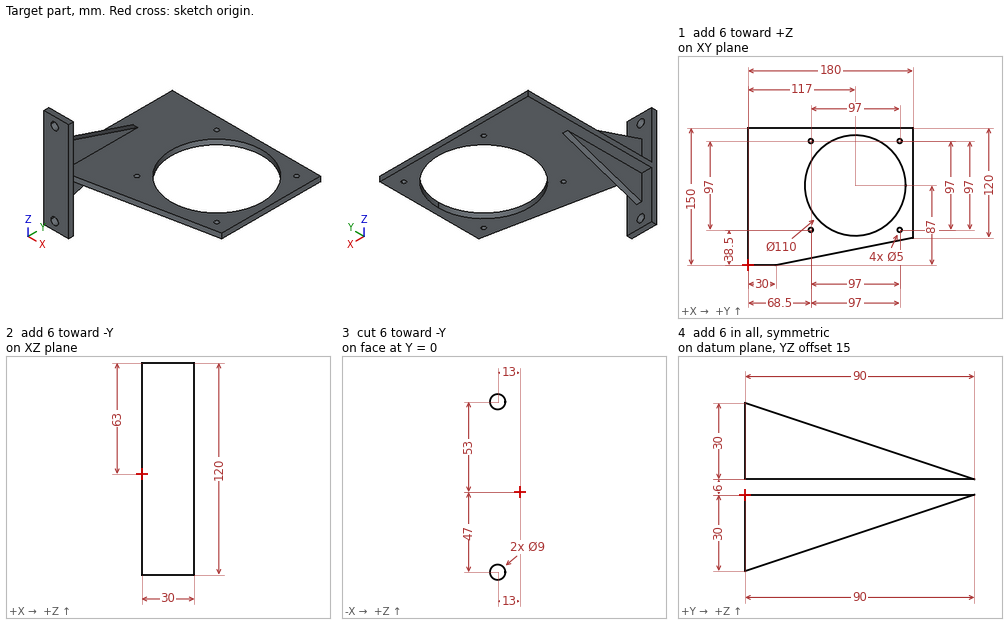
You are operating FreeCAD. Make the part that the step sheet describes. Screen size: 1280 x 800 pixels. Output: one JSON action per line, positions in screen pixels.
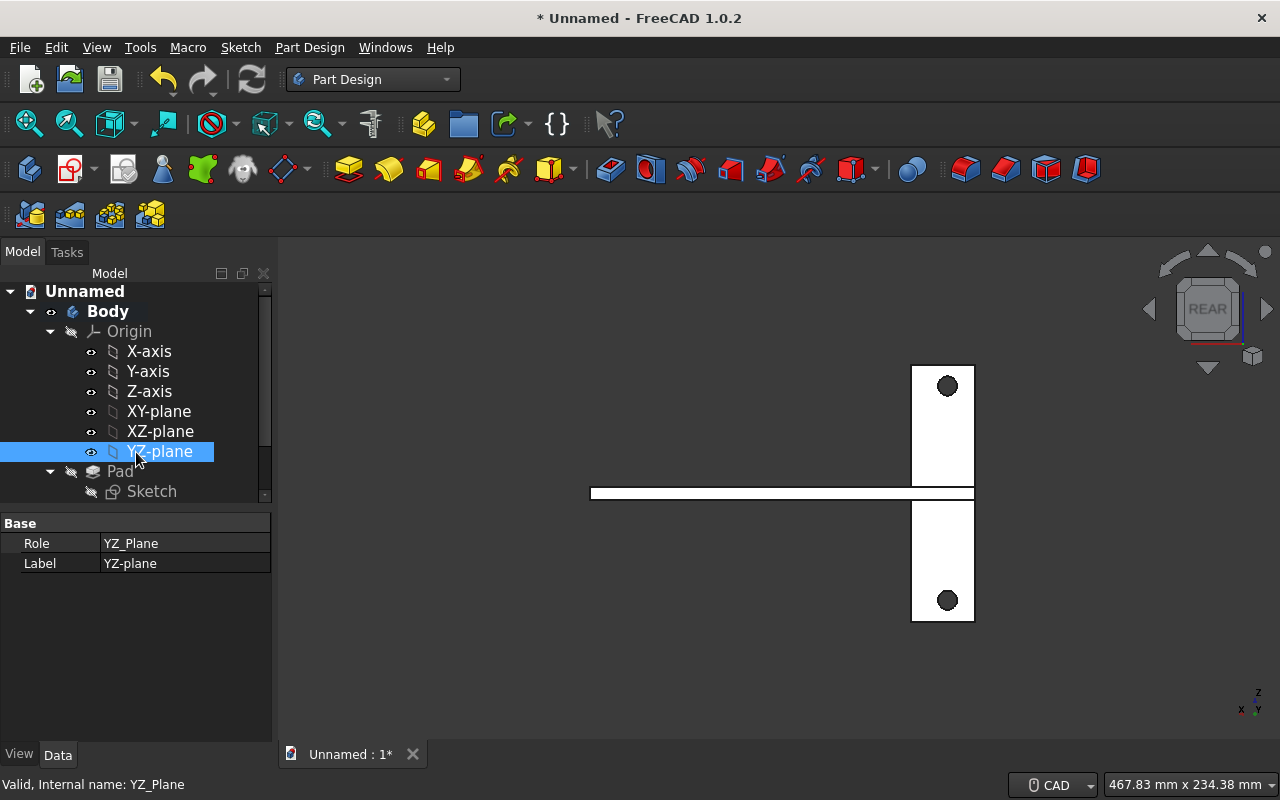
{"action": "left_click", "coordinate": [284, 170]}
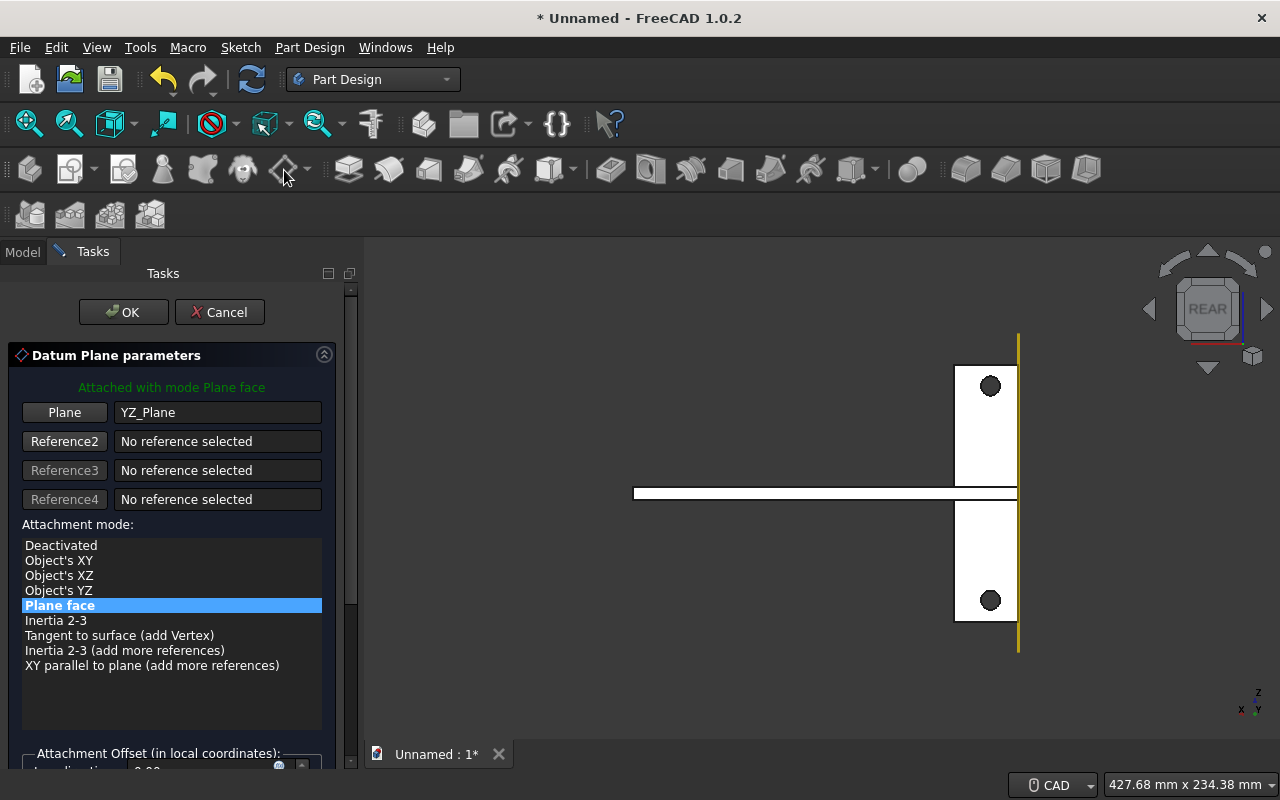
{"action": "scroll", "coordinate": [351, 526], "scroll_direction": "down", "scroll_amount": 3}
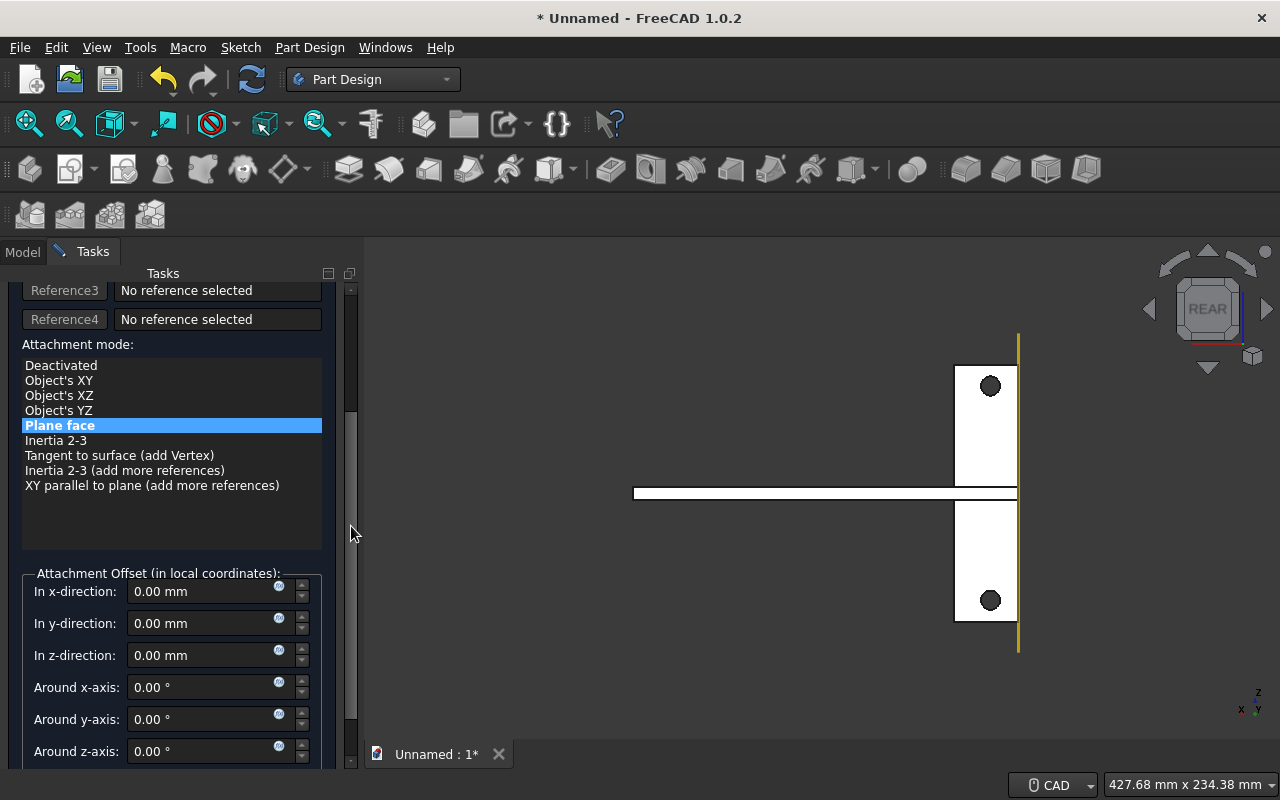
{"action": "triple_click", "coordinate": [210, 655]}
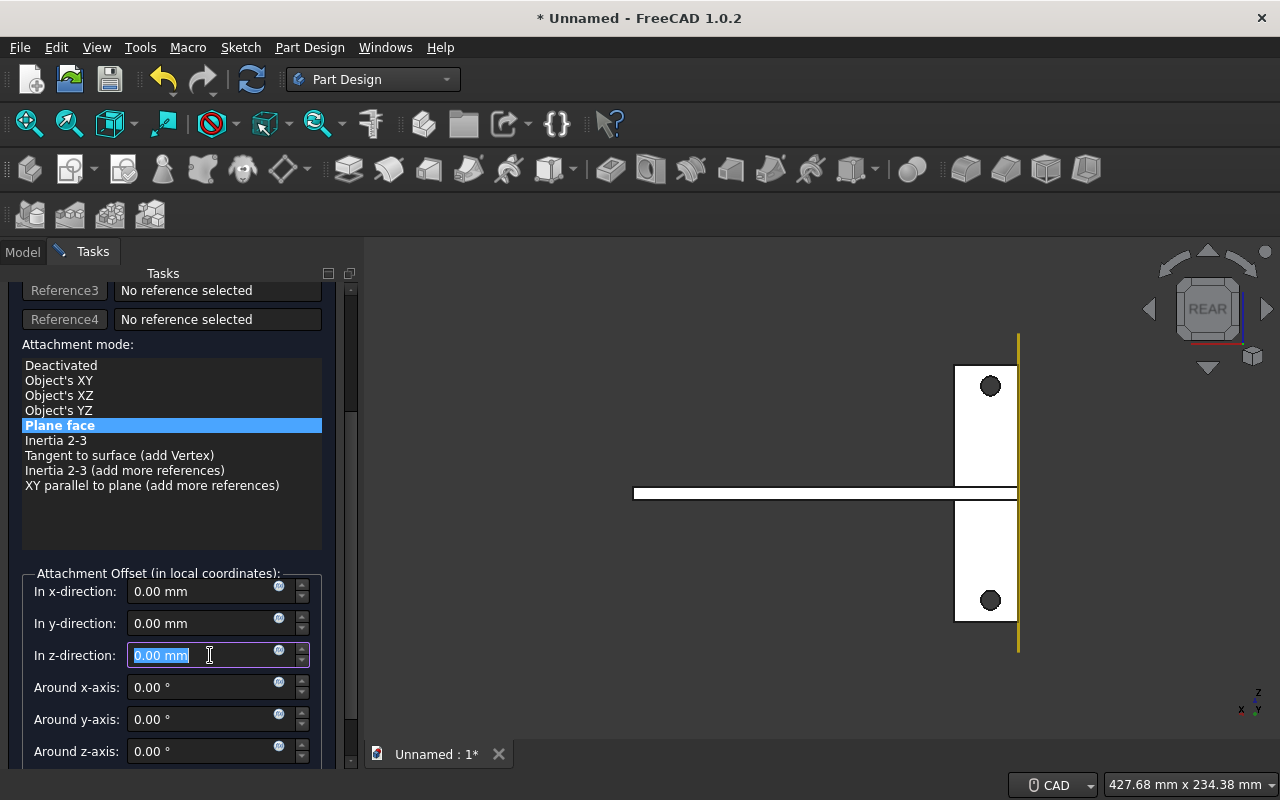
{"action": "type", "text": "15"}
{"action": "key", "text": "Tab"}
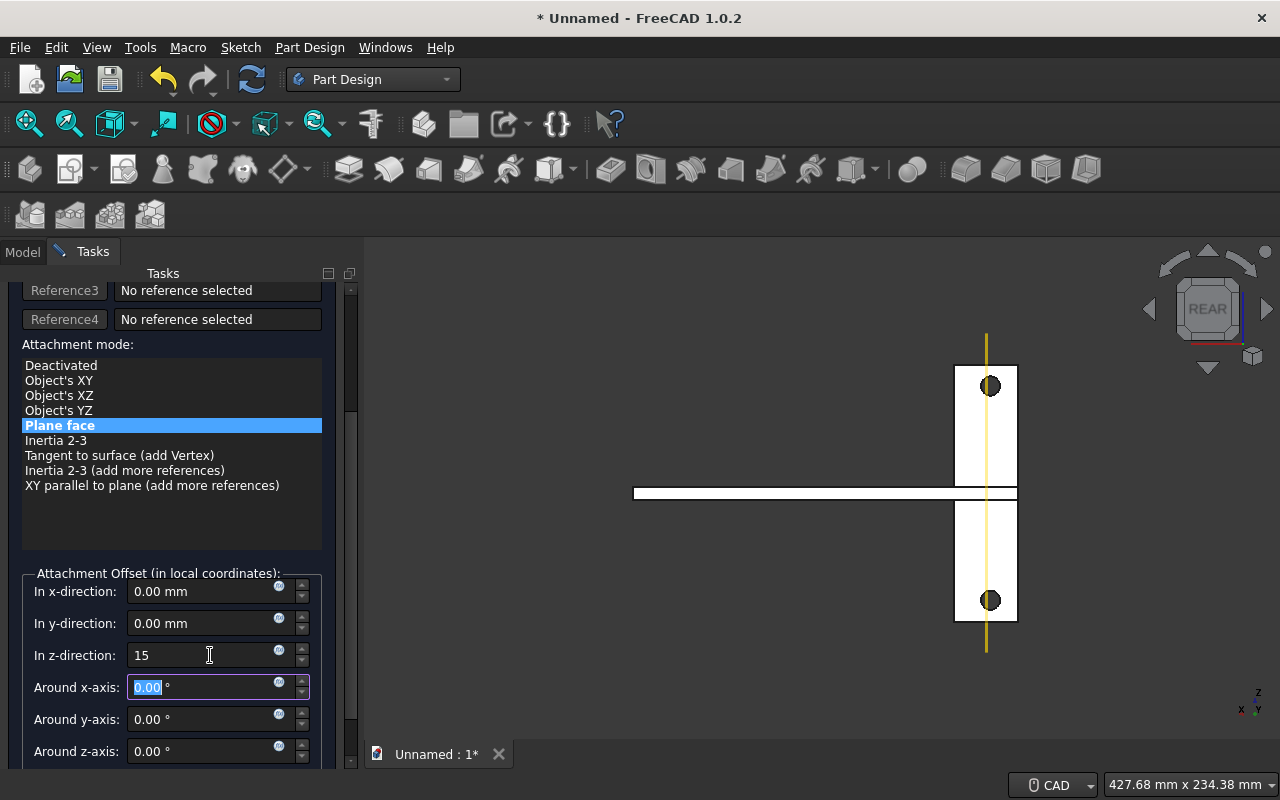
{"action": "scroll", "coordinate": [351, 526], "scroll_direction": "up", "scroll_amount": 4}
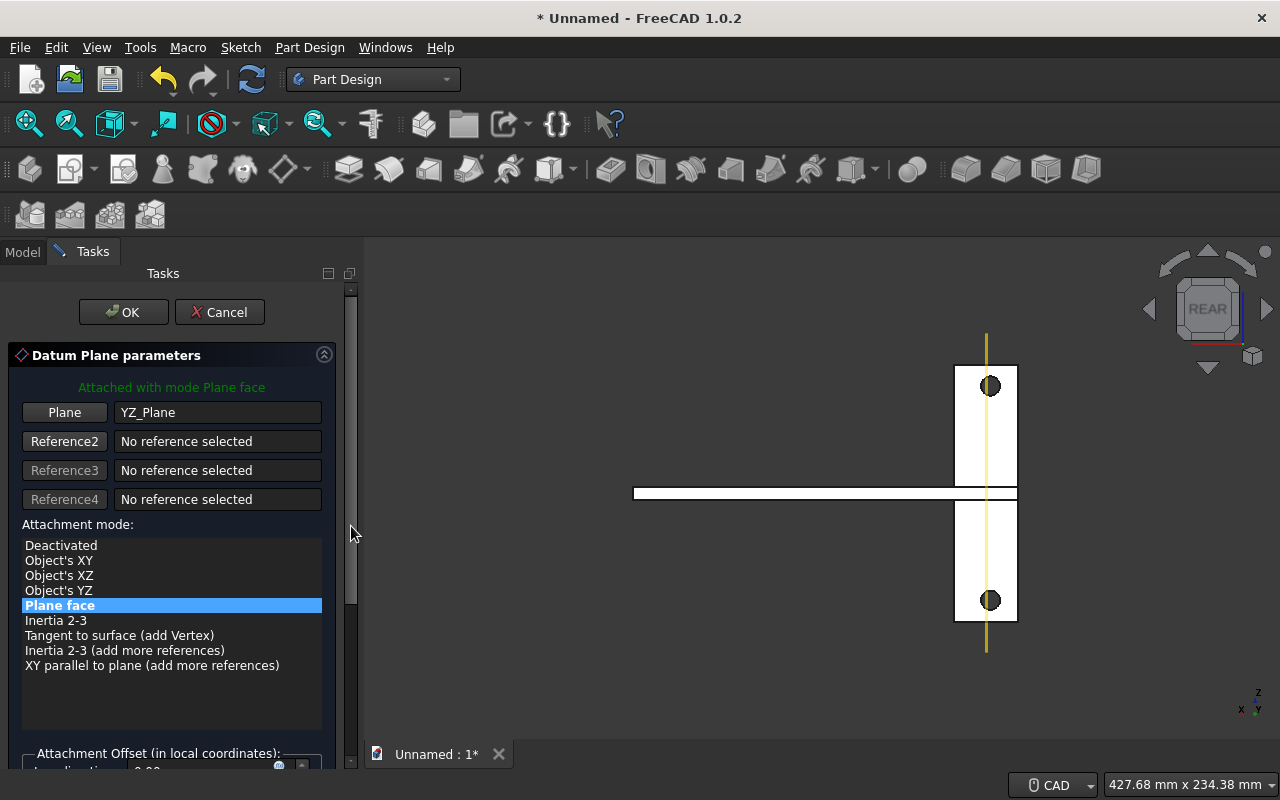
{"action": "left_click", "coordinate": [124, 312]}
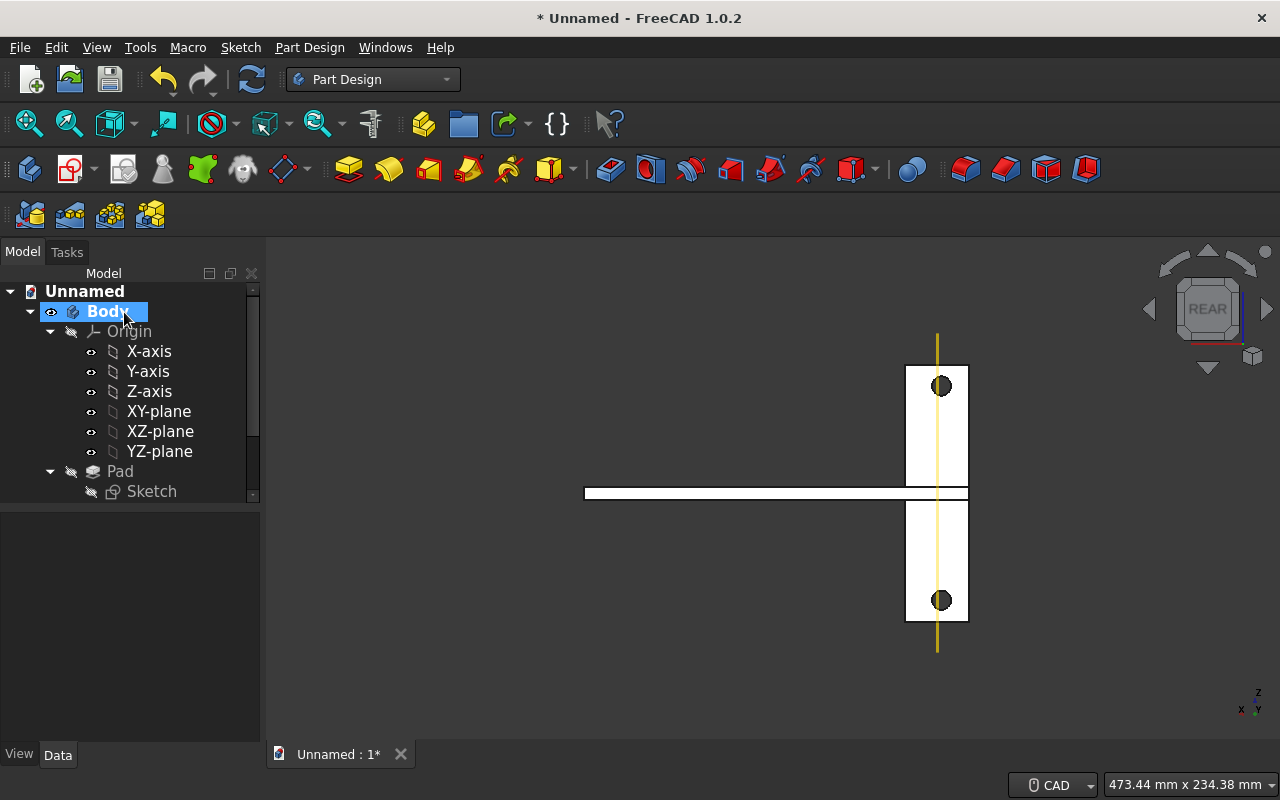
{"action": "scroll", "coordinate": [100, 387], "scroll_direction": "down", "scroll_amount": 3}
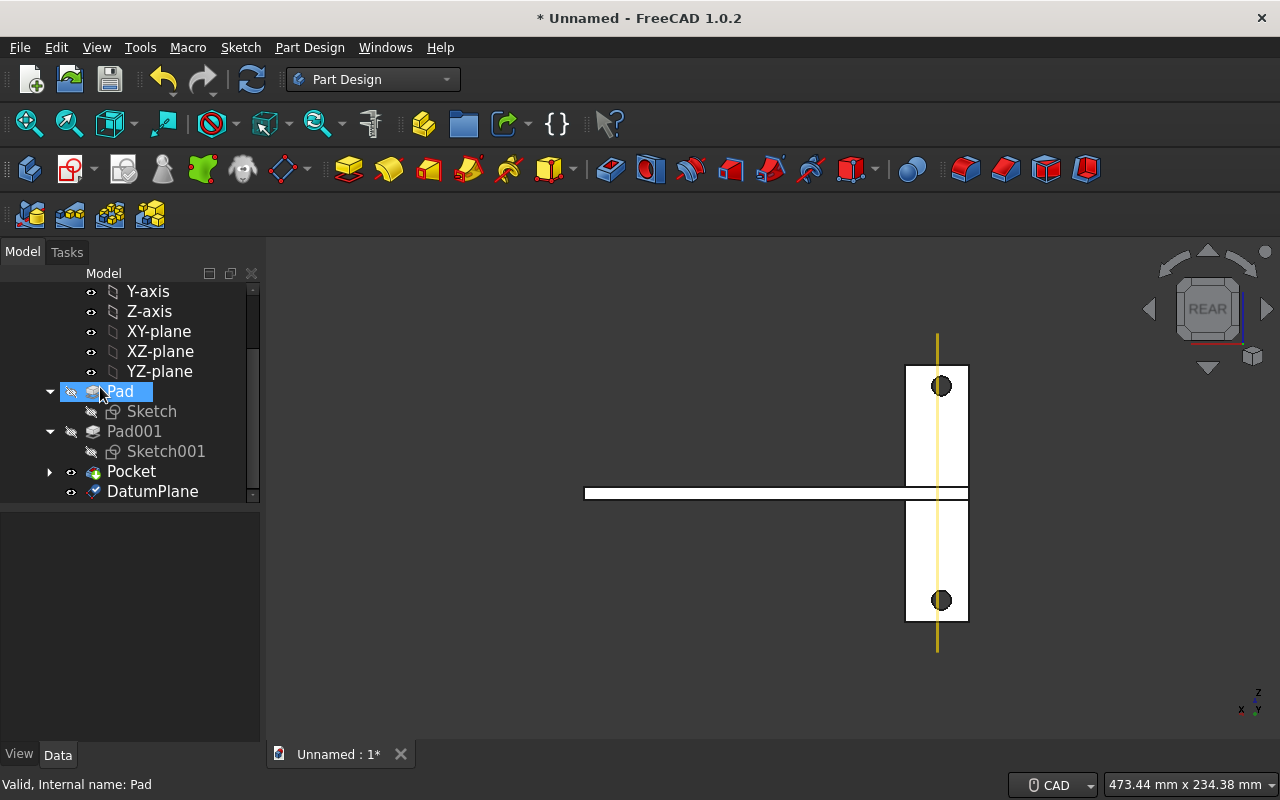
{"action": "left_click", "coordinate": [116, 492]}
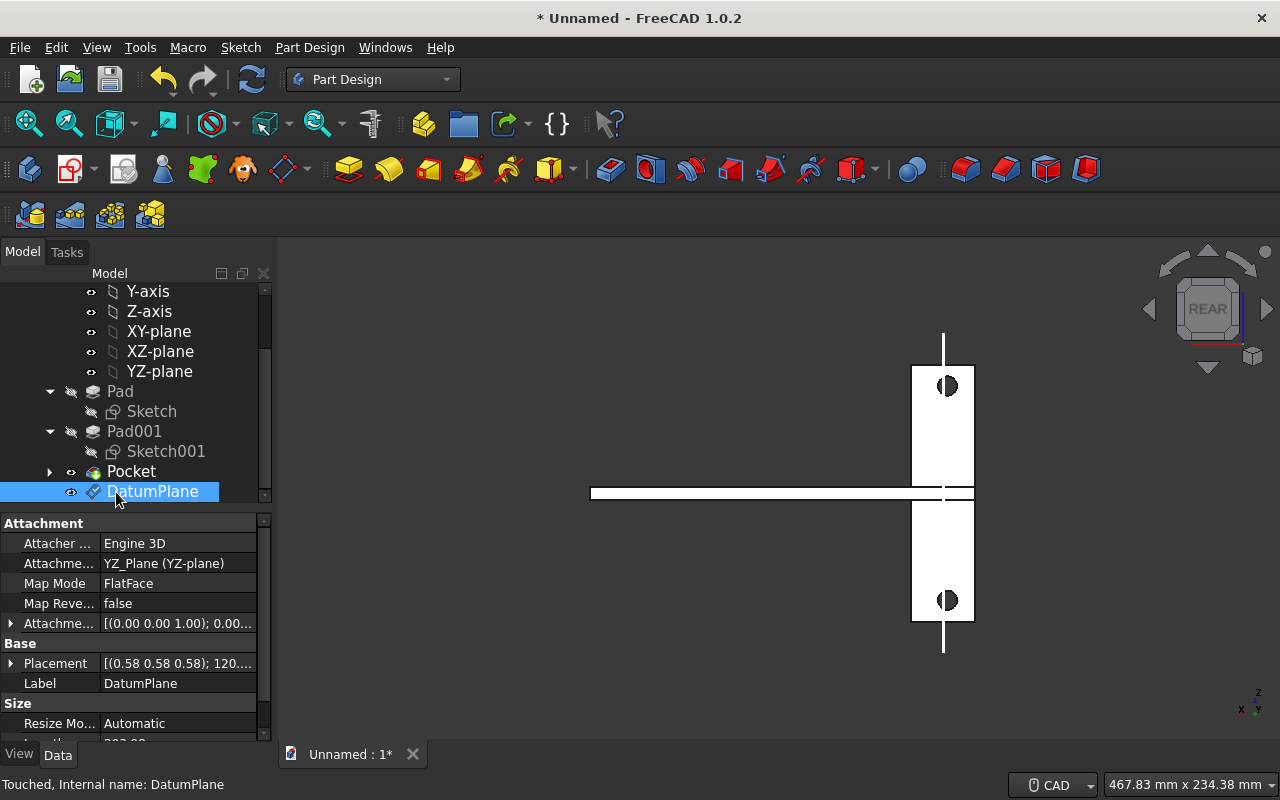
{"action": "left_click", "coordinate": [70, 170]}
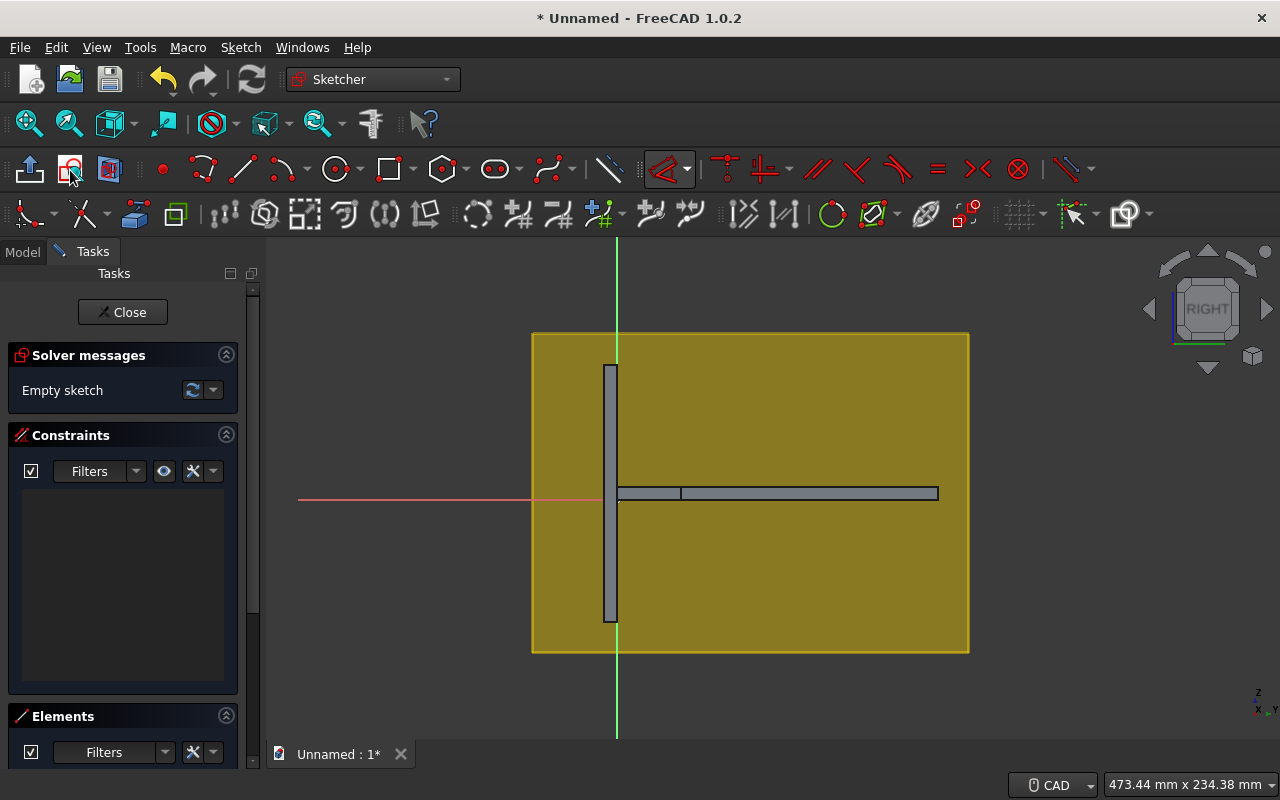
{"action": "key", "text": "q s"}